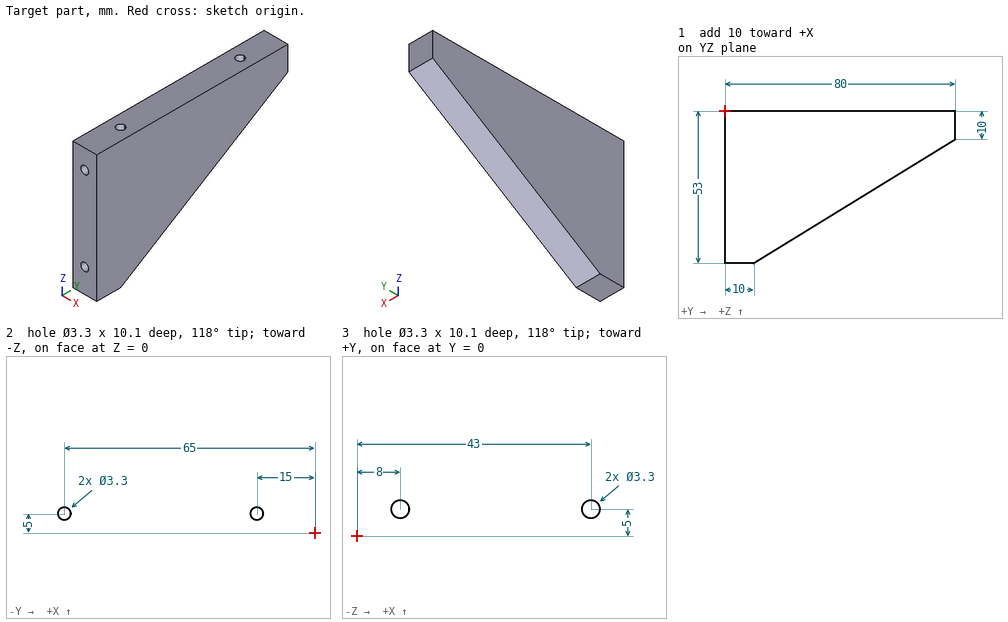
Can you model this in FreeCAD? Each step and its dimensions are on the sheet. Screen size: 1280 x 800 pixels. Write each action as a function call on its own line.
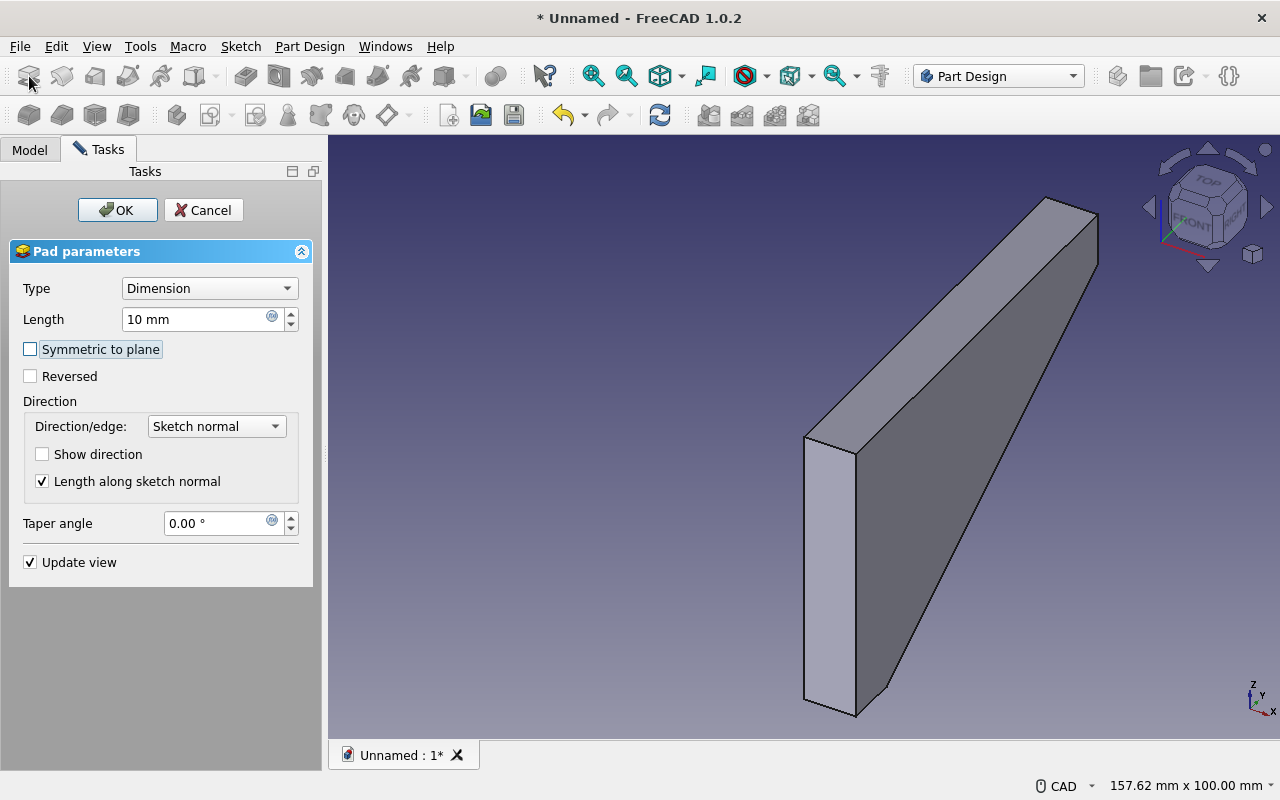
click(118, 210)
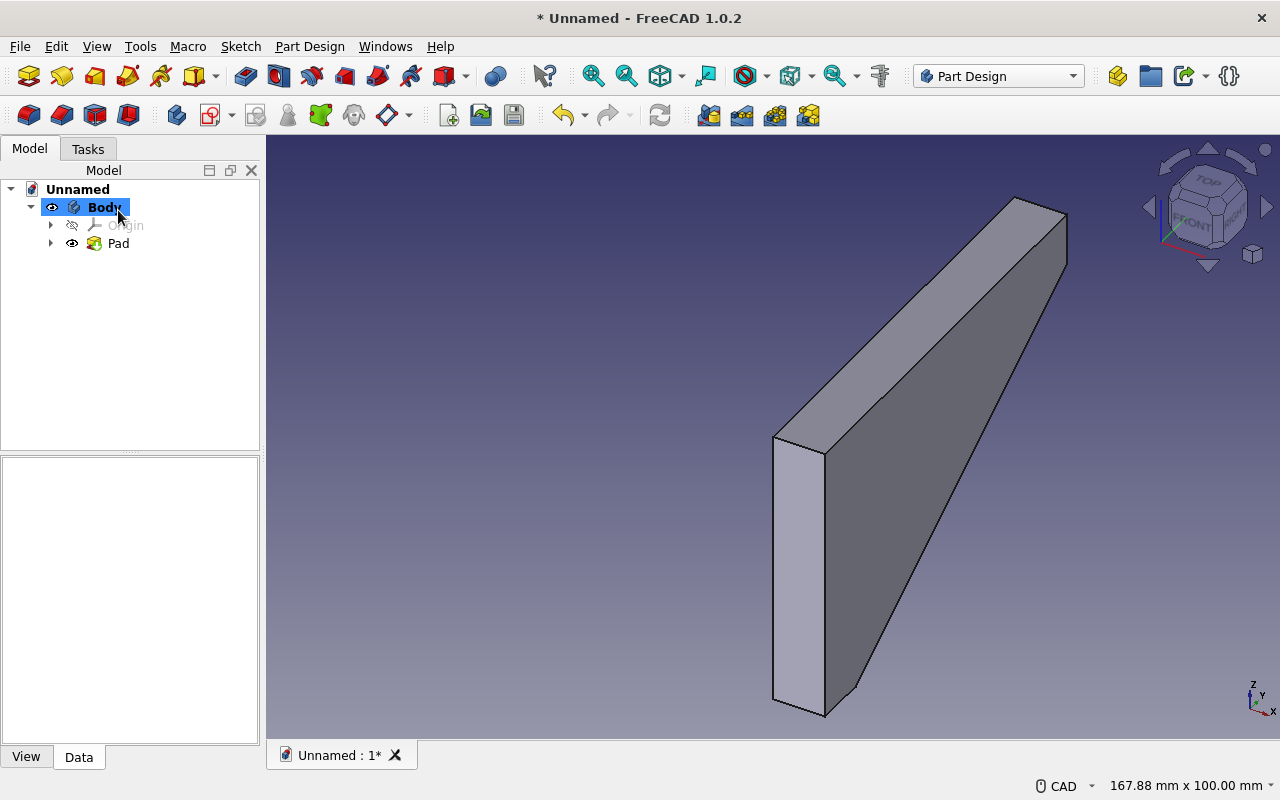
click(1023, 222)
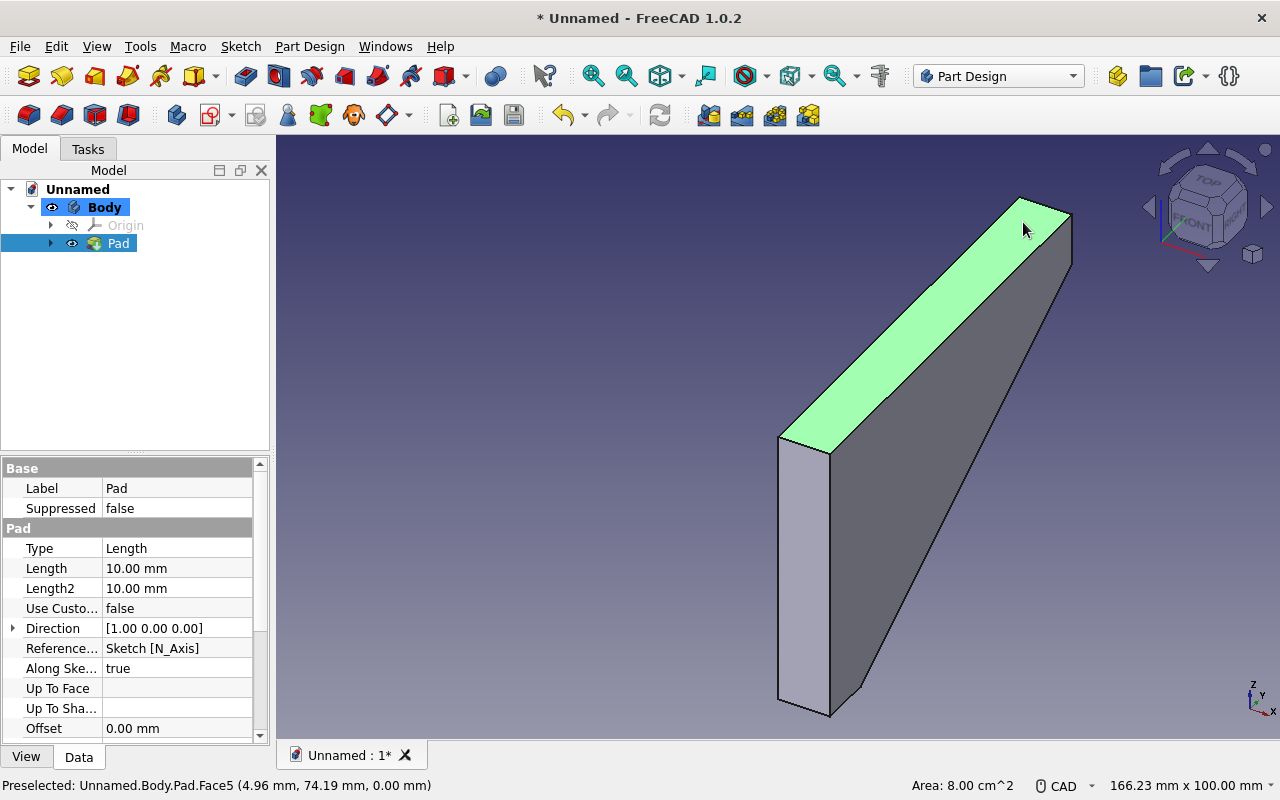
click(210, 116)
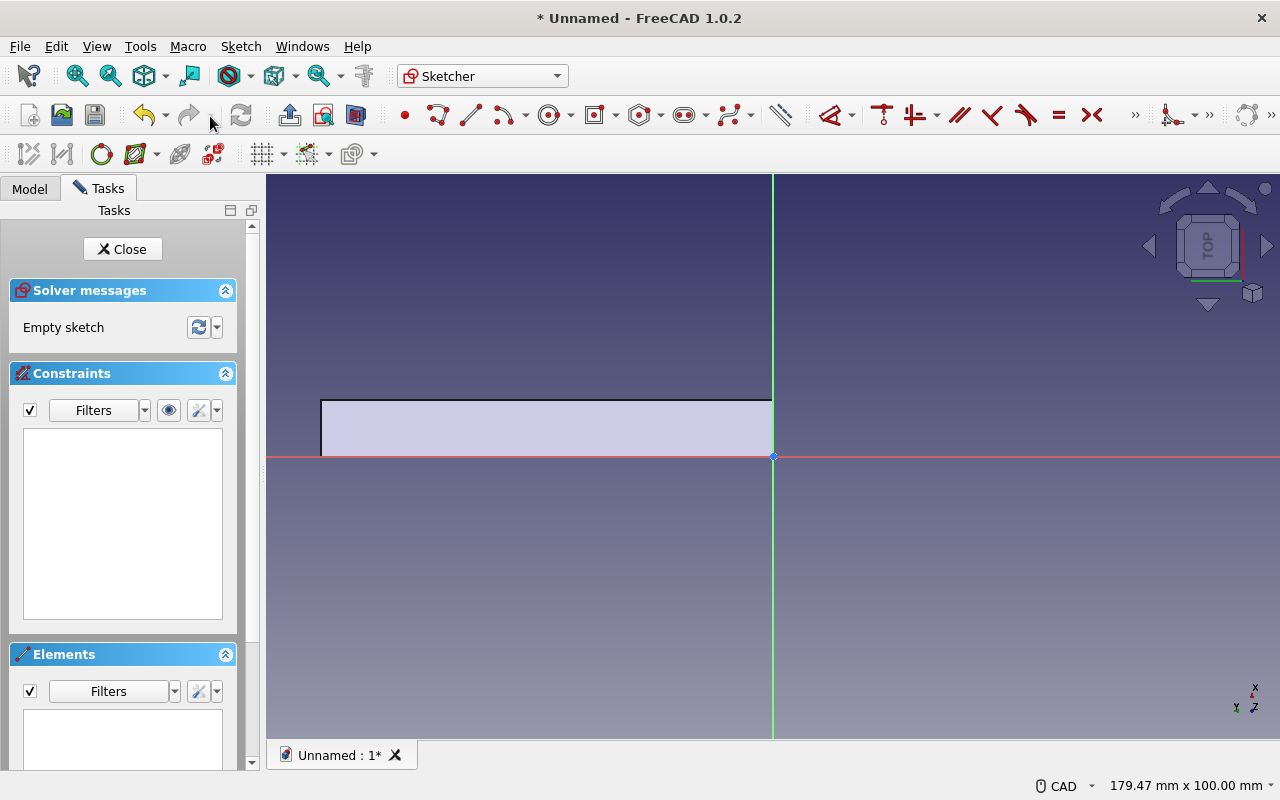
scroll(341, 400, up, 2)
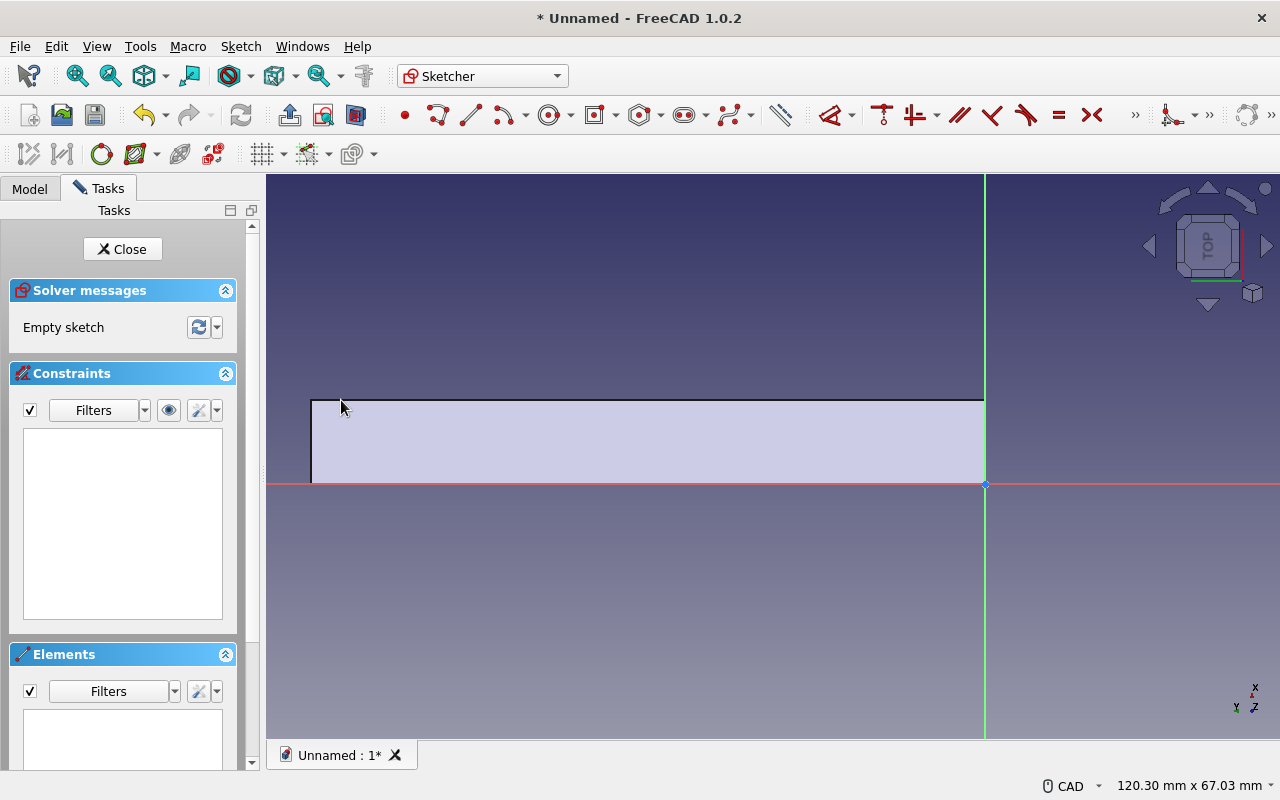
click(548, 116)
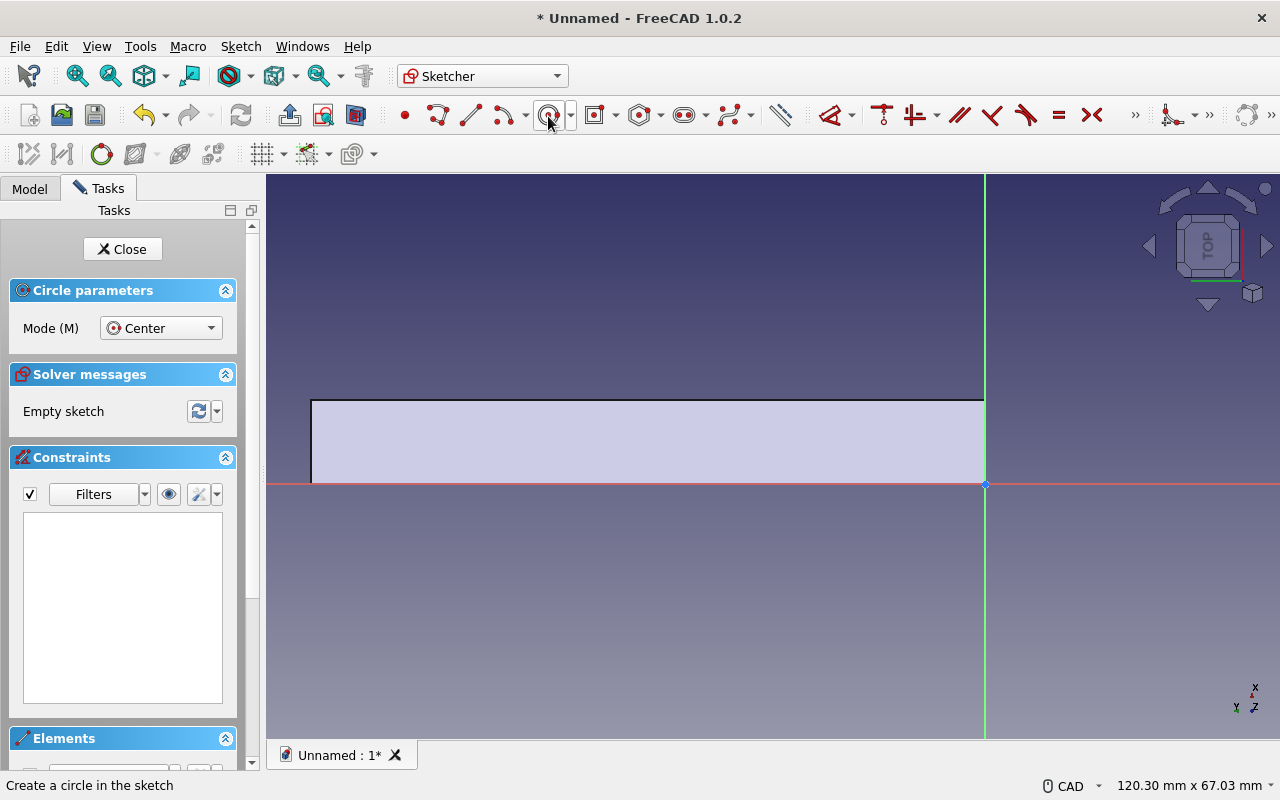
scroll(438, 442, up, 3)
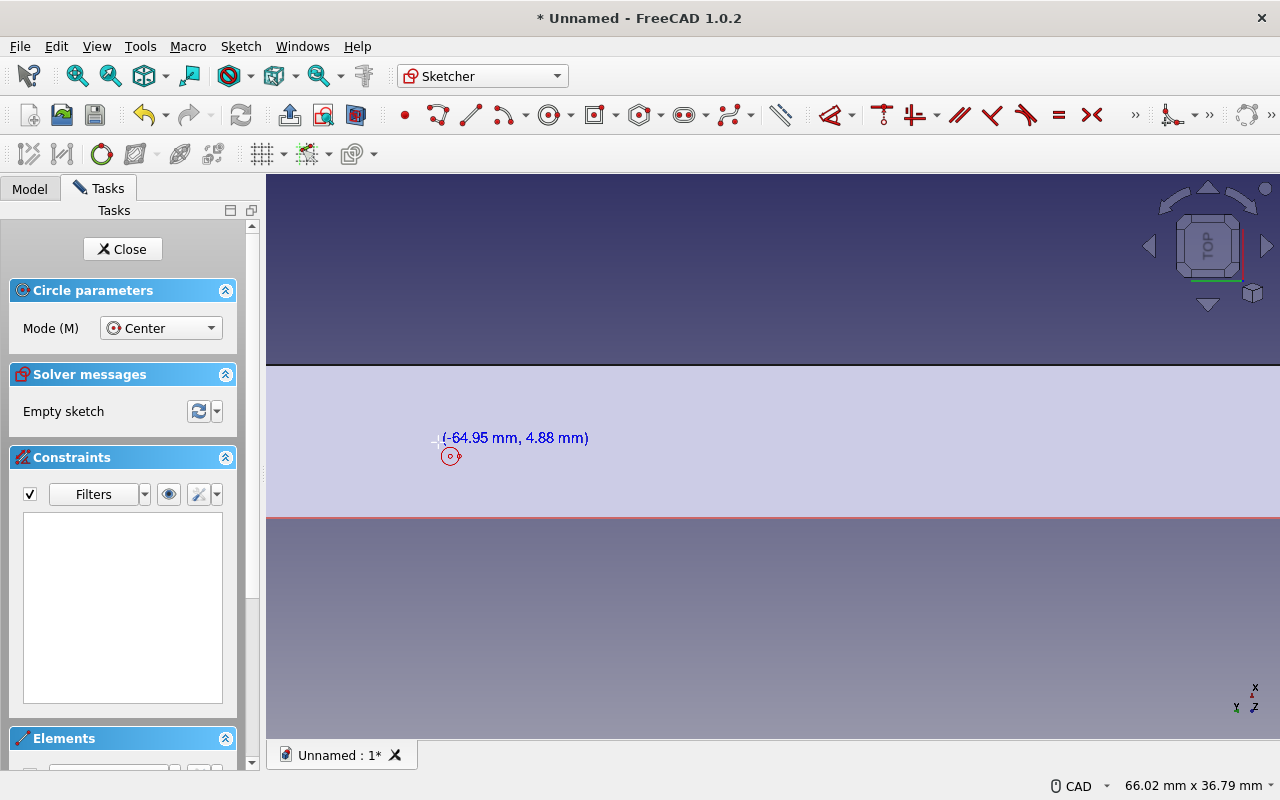
click(437, 442)
move(455, 424)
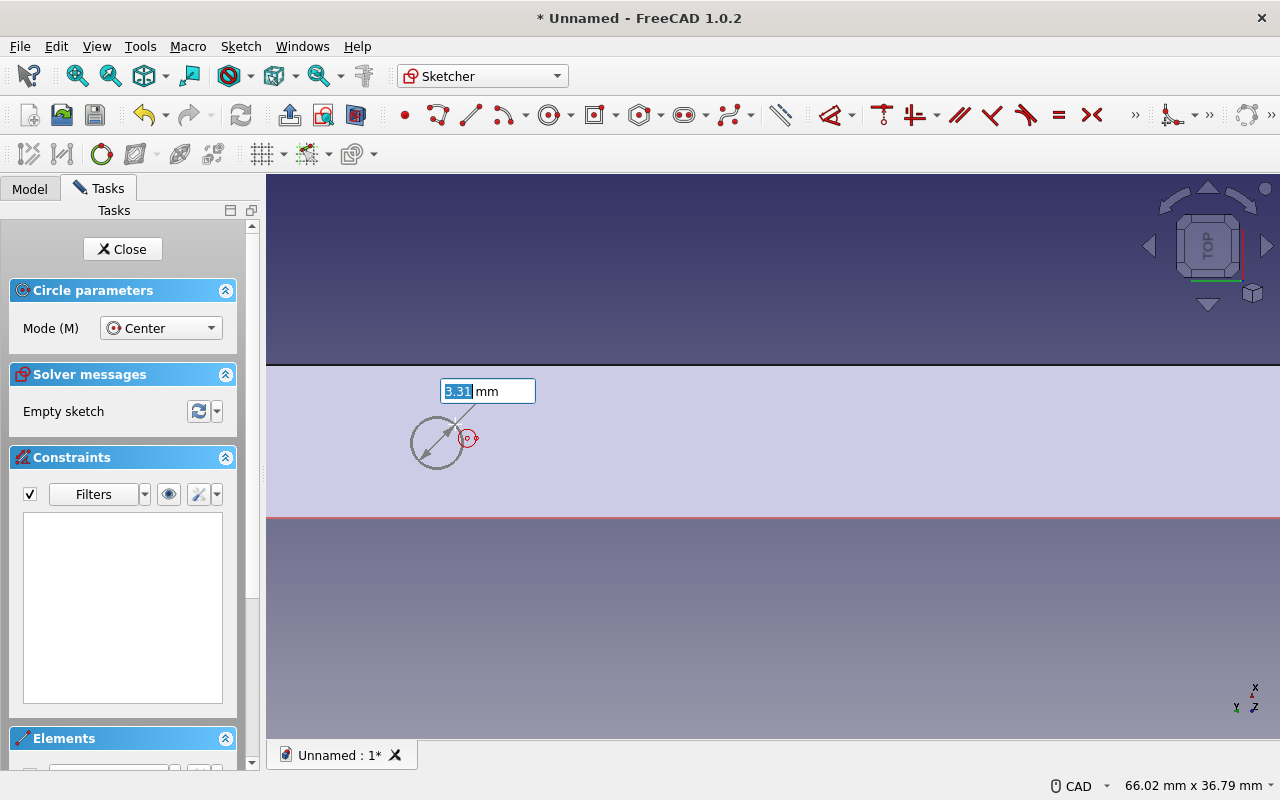
text(3.3)
key(Return)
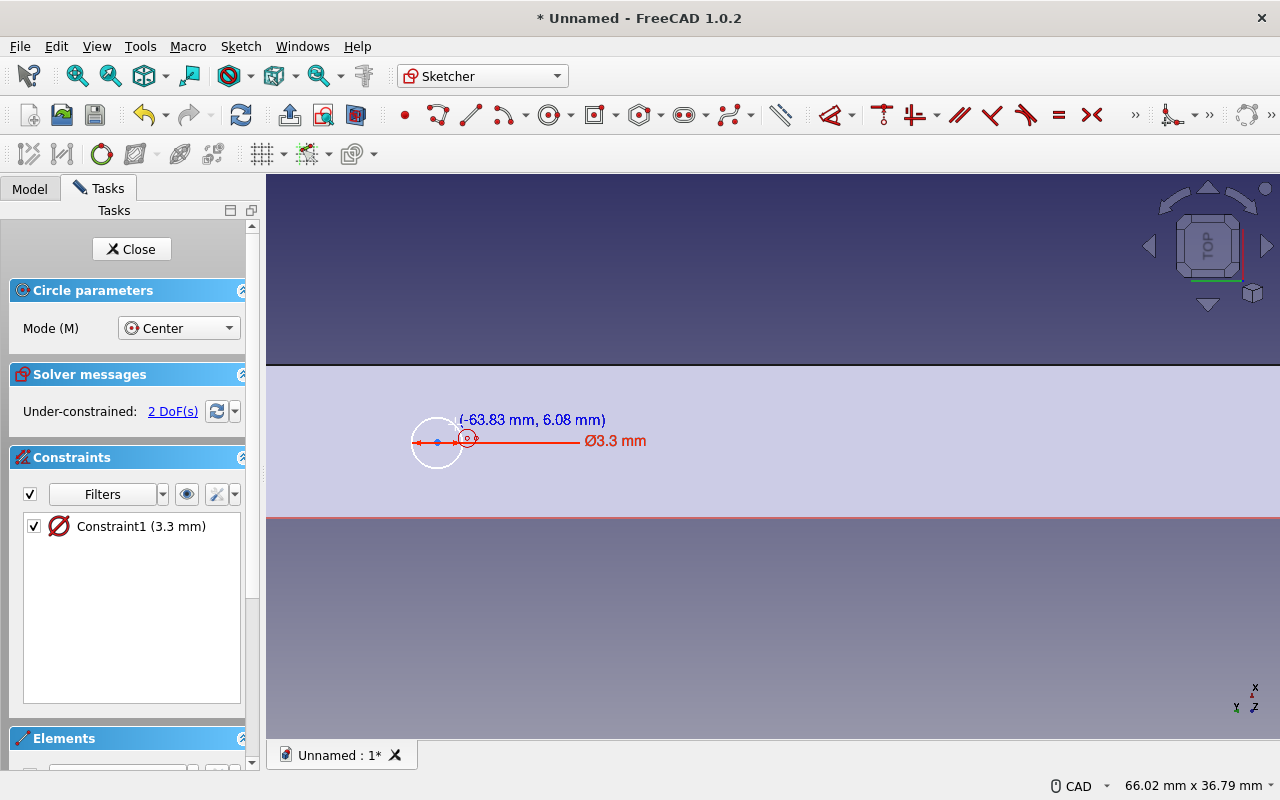
scroll(438, 443, down, 3)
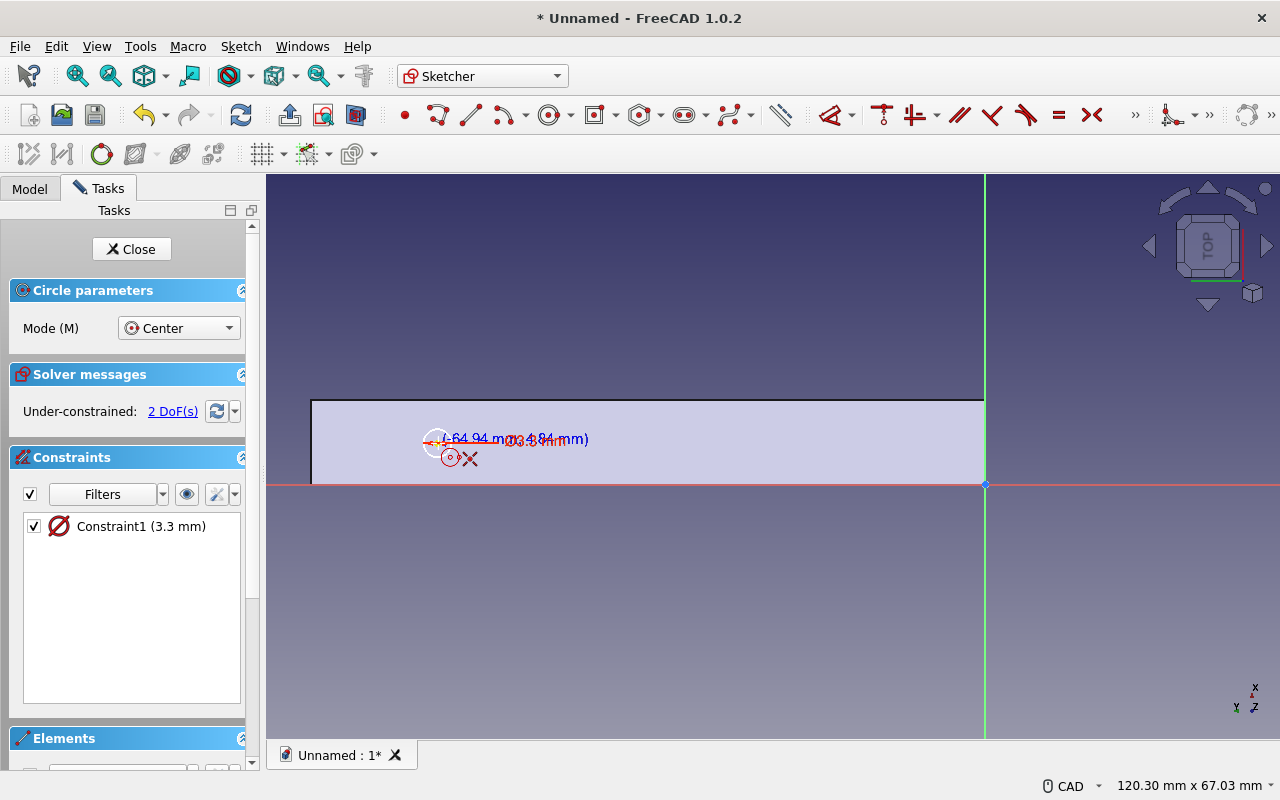
scroll(859, 442, up, 3)